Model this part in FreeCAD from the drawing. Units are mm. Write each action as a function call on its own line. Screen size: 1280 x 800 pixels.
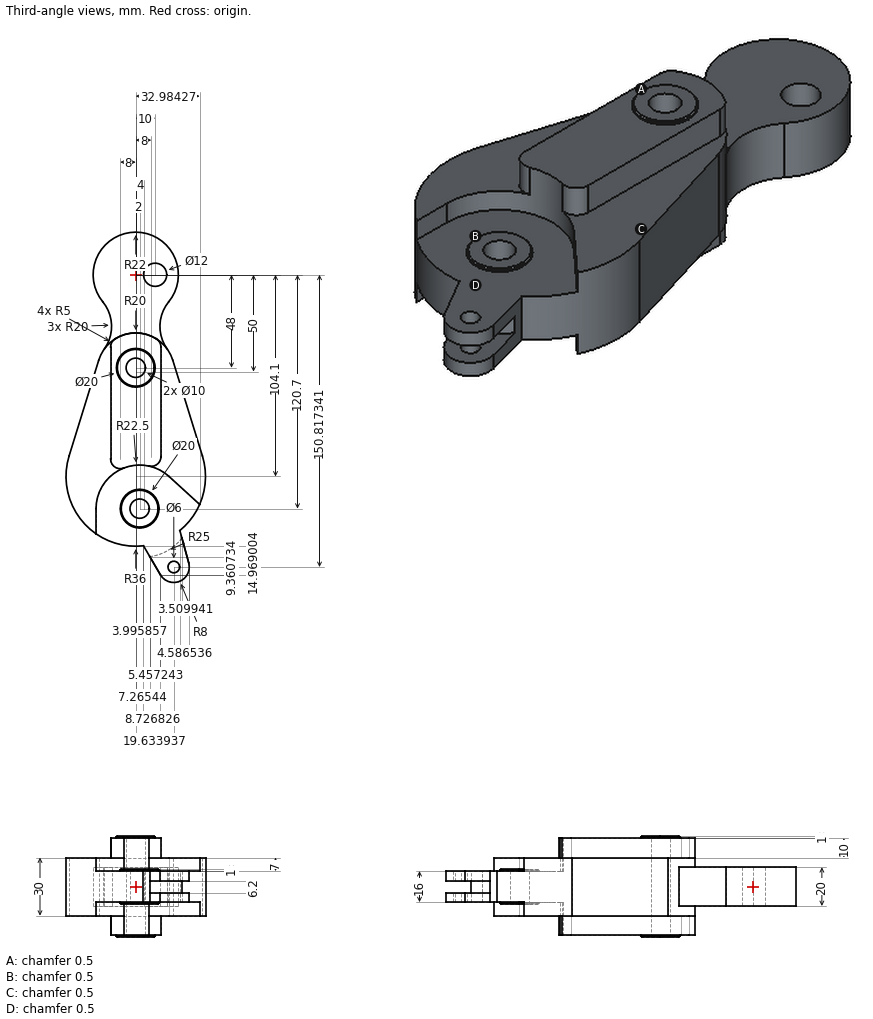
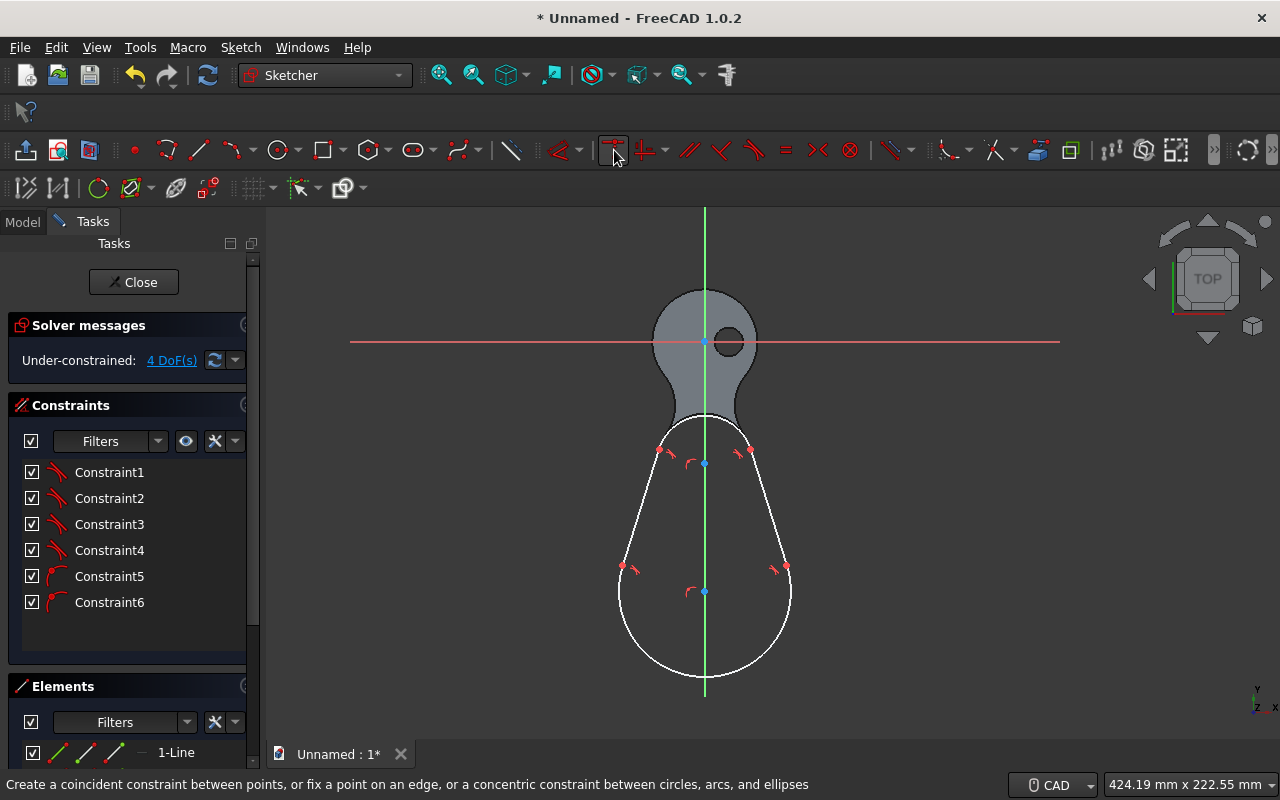
click(558, 150)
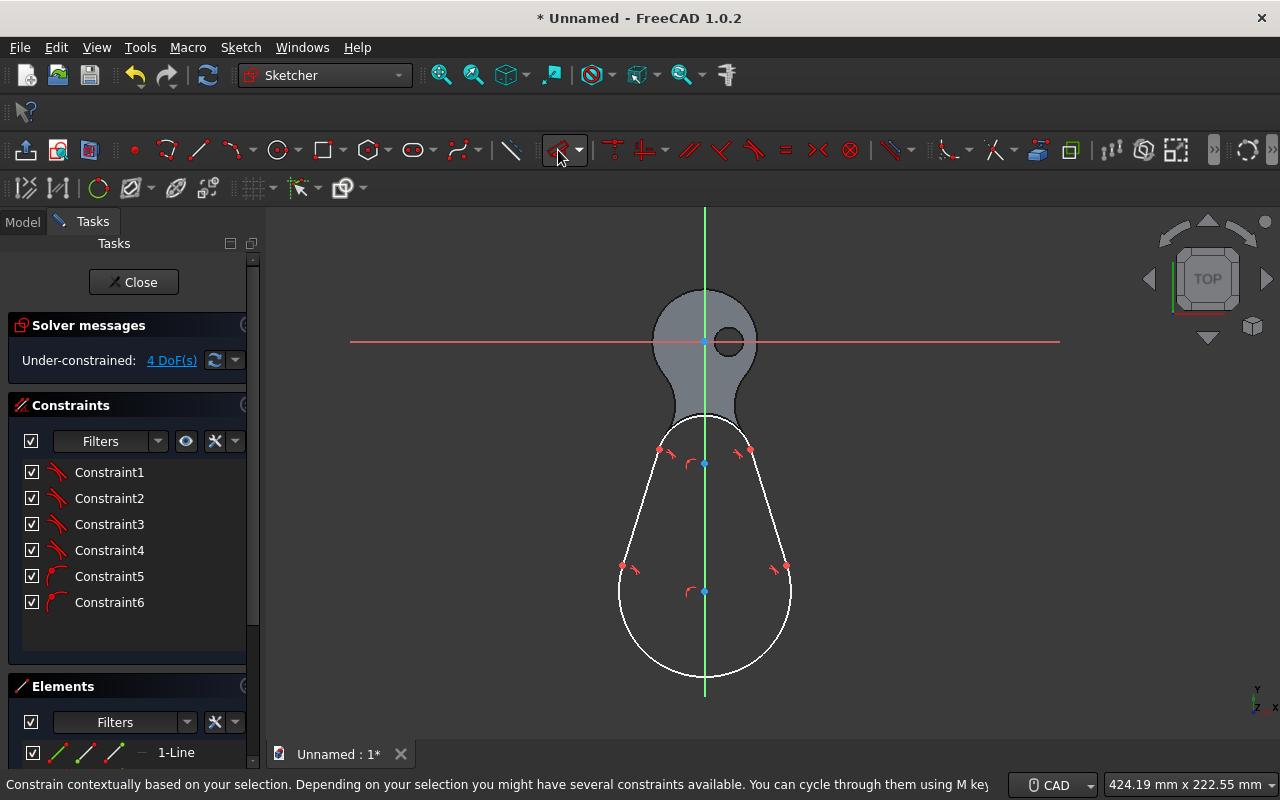
click(646, 654)
click(624, 677)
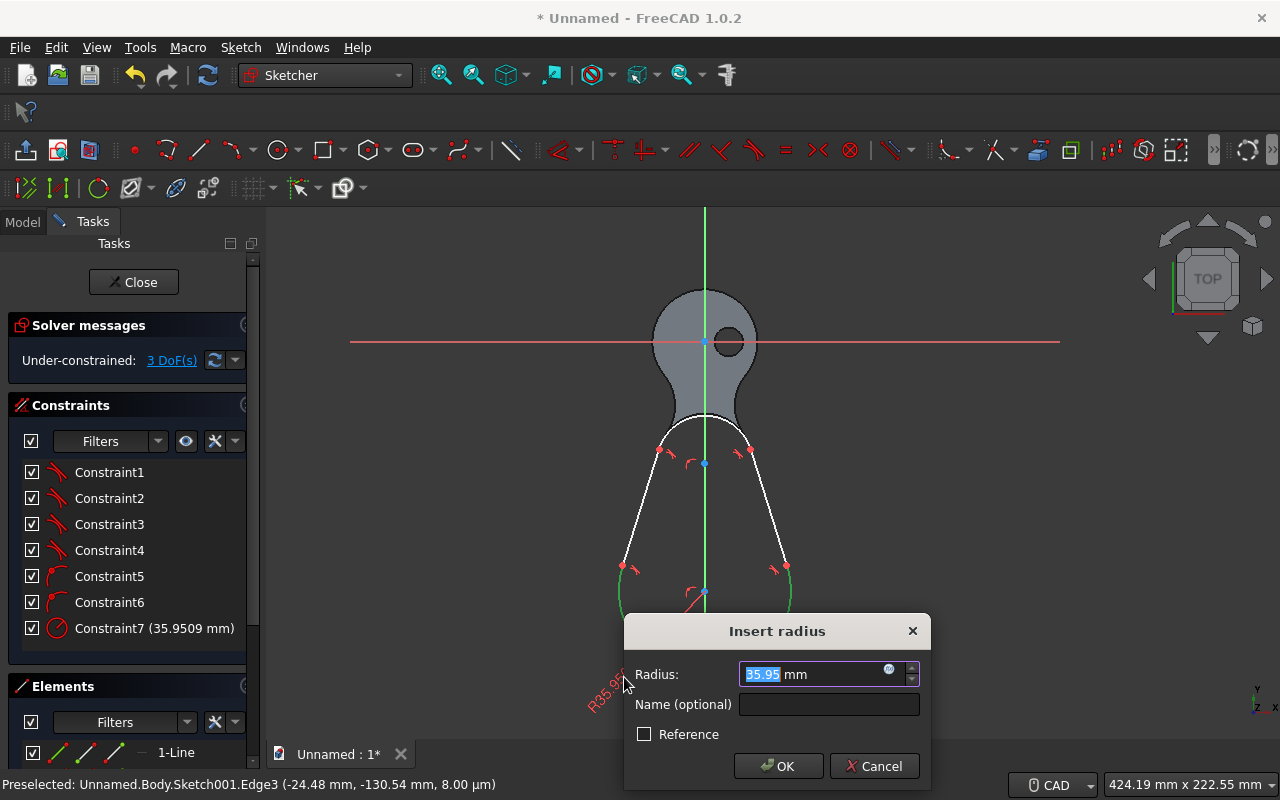
text(36)
key(Return)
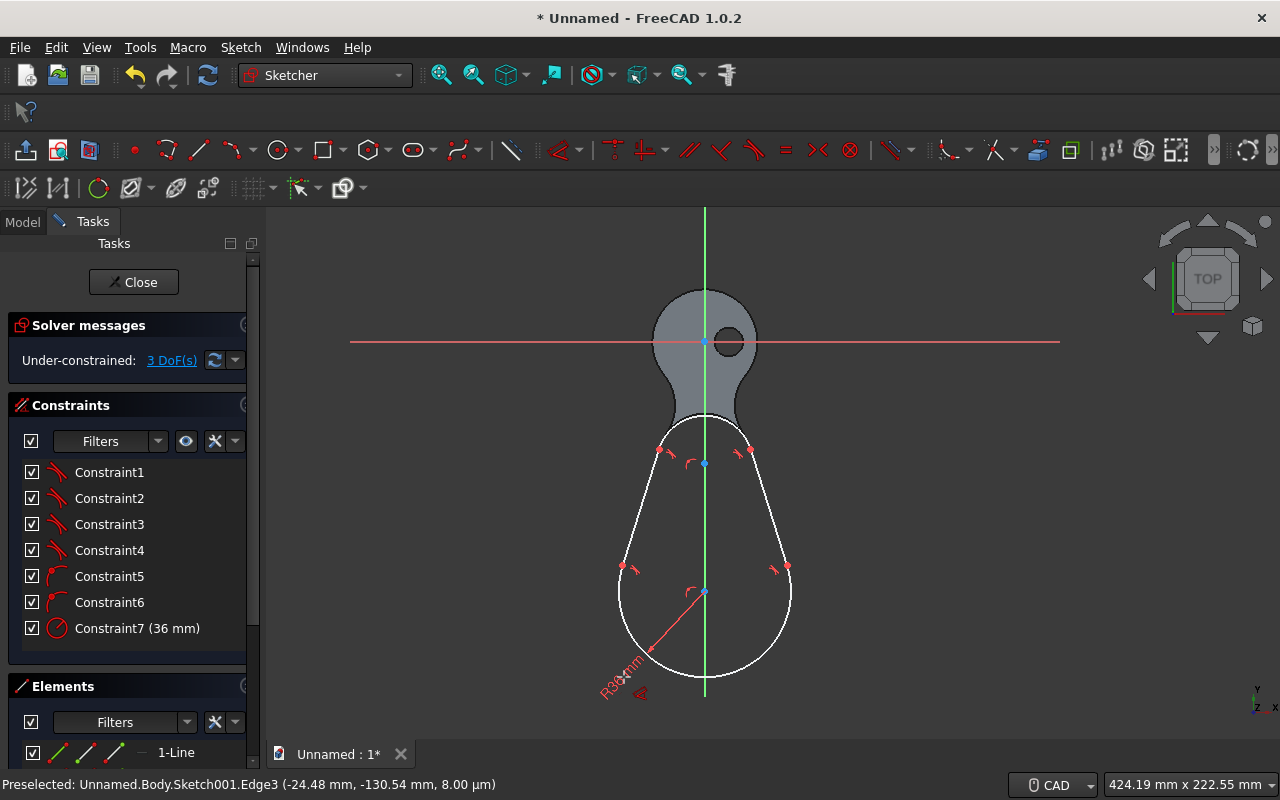
click(728, 422)
click(743, 394)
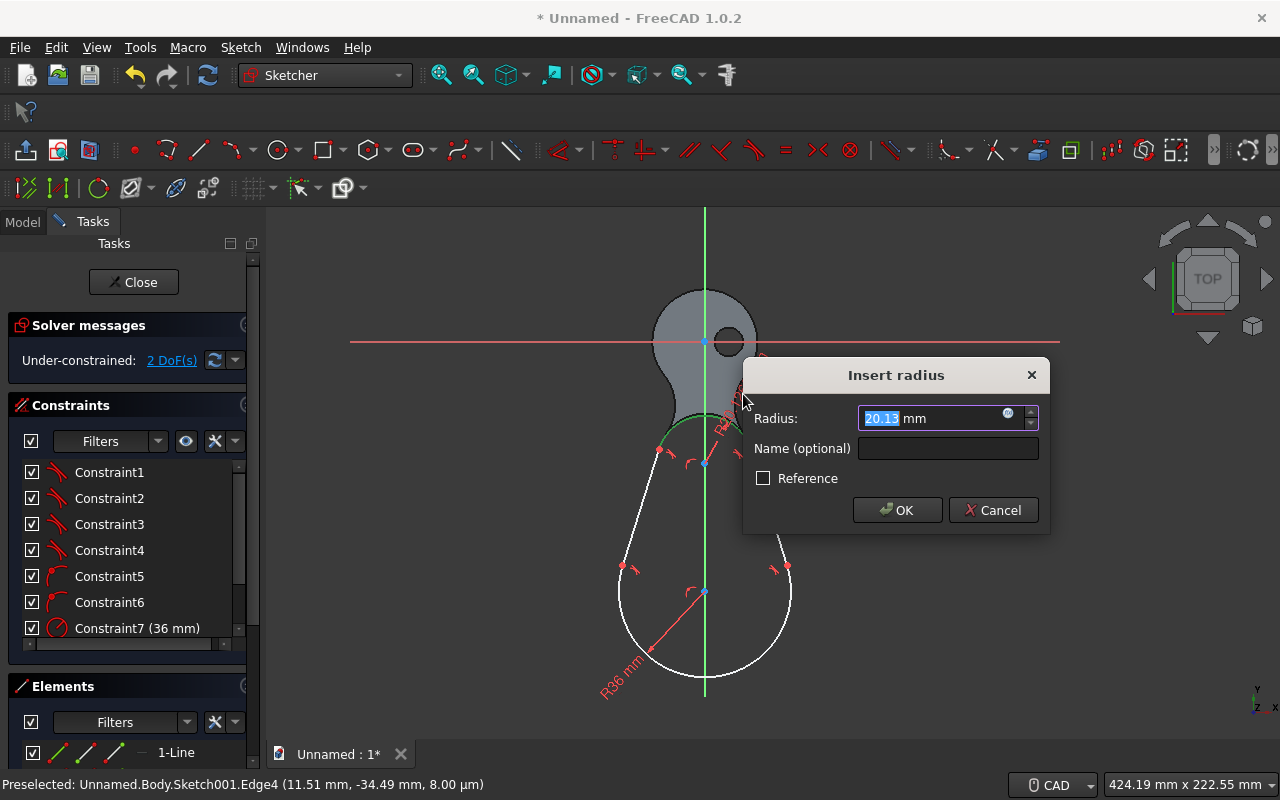
text(20)
key(Return)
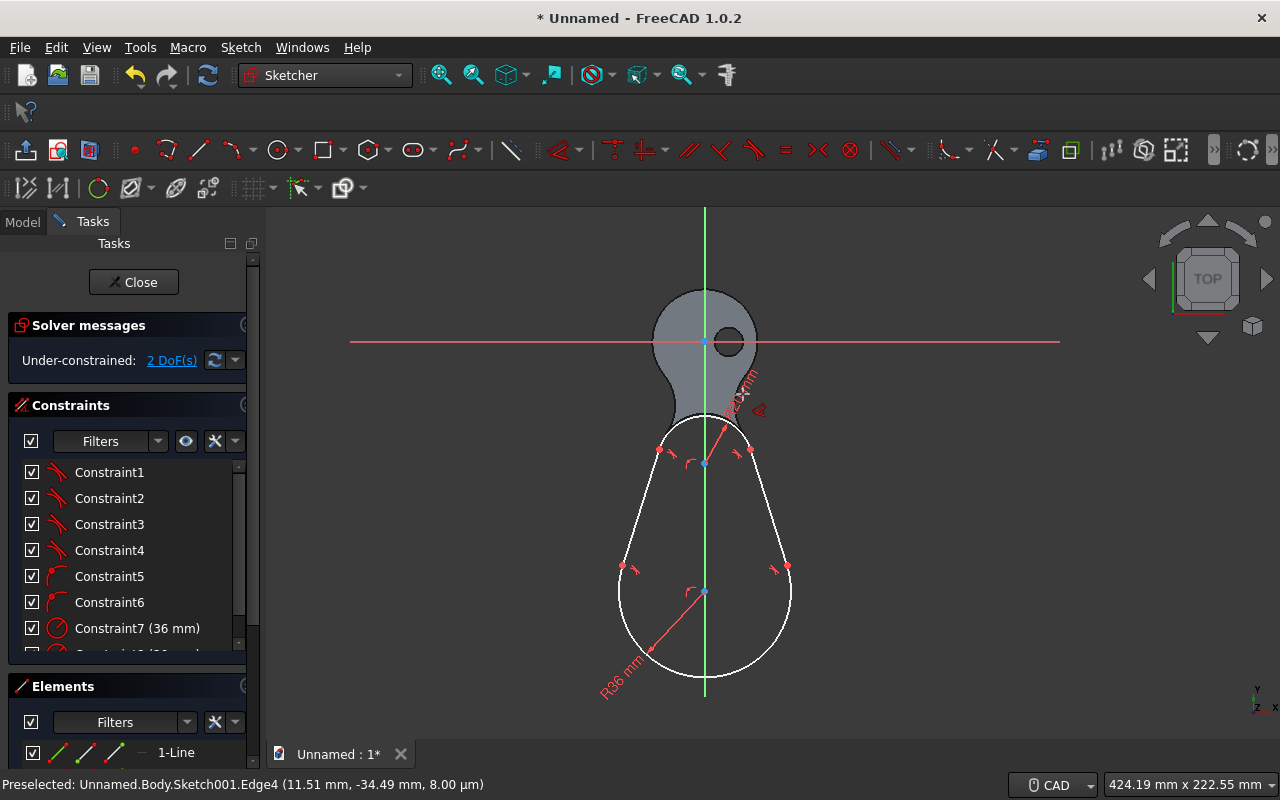
click(705, 464)
click(739, 360)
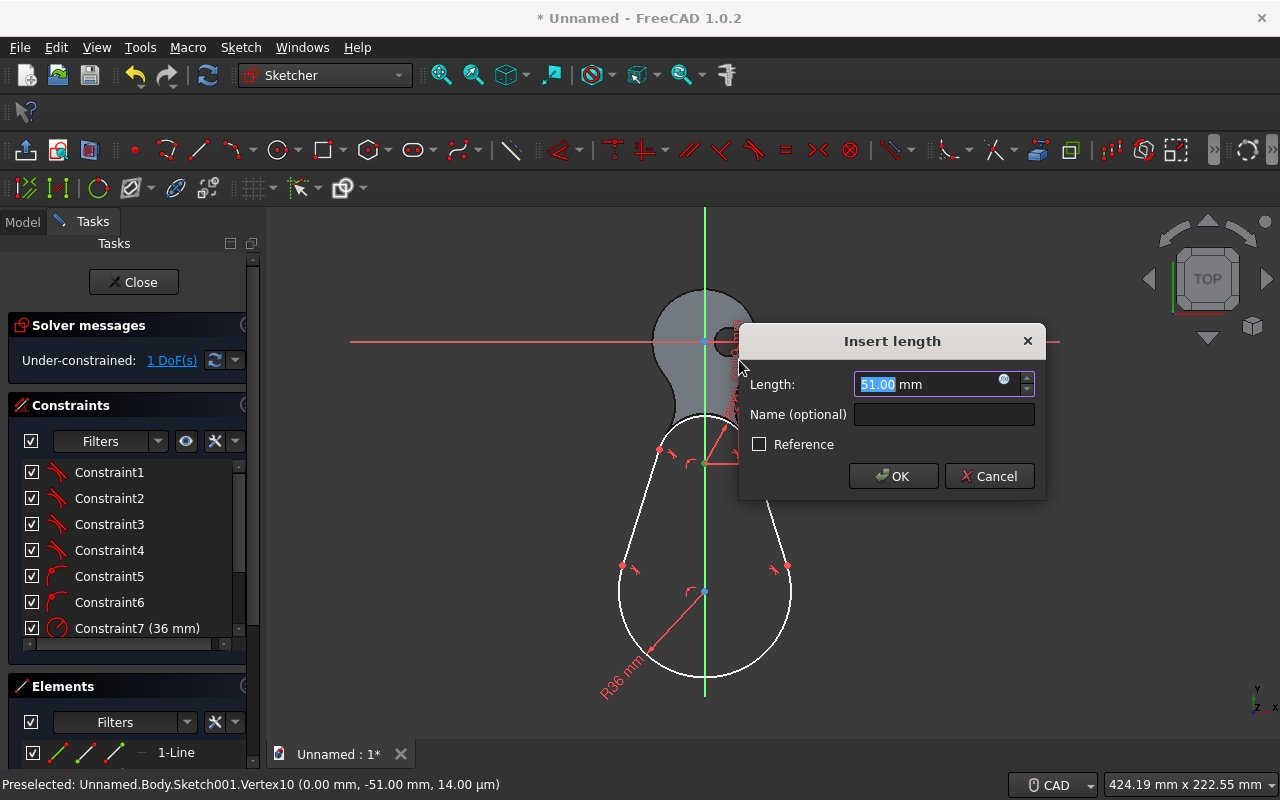
text(50)
key(Return)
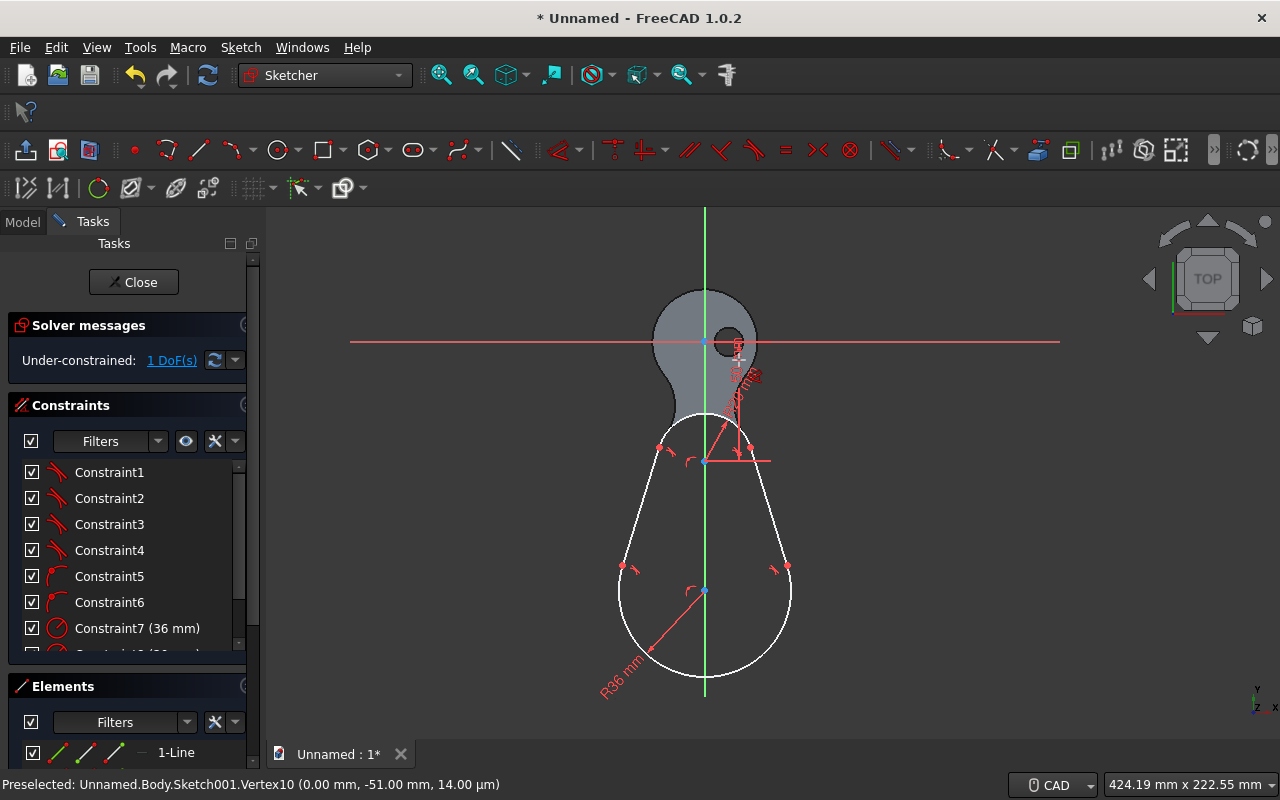
click(705, 591)
click(739, 466)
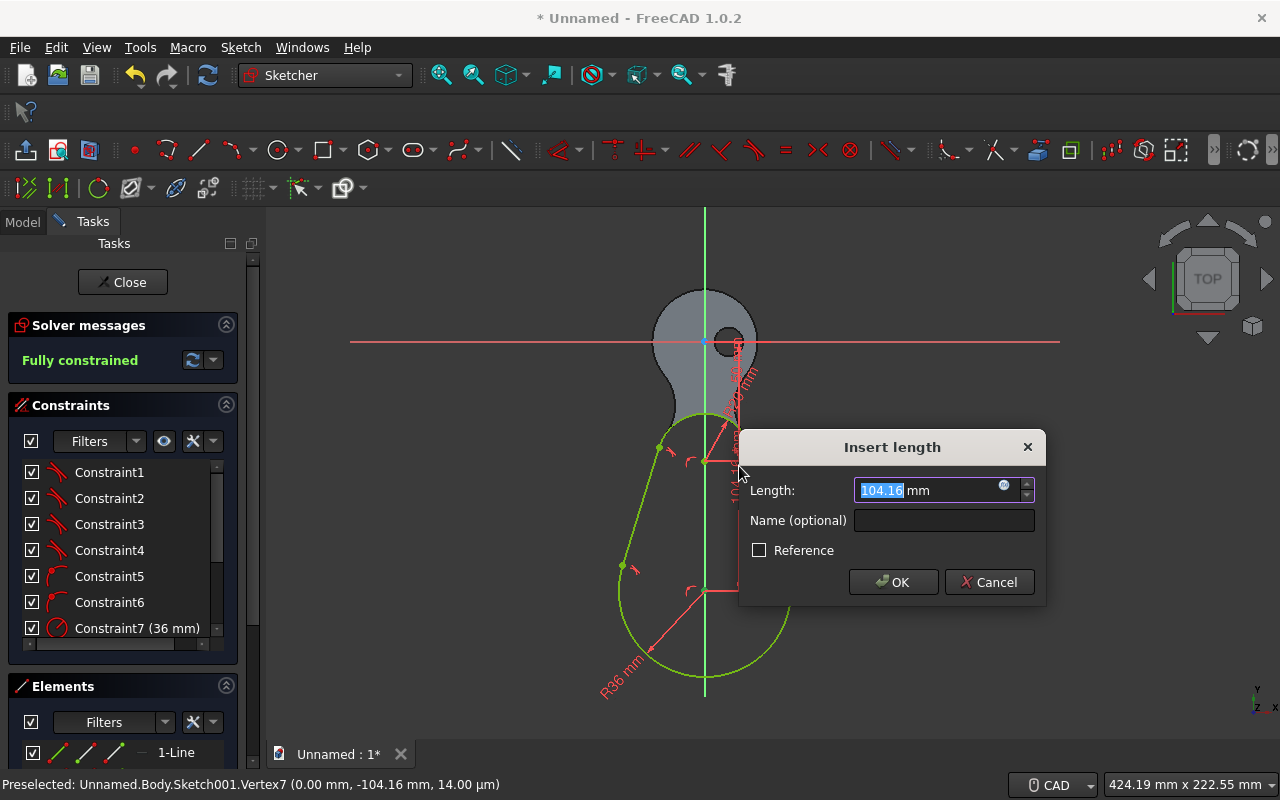
text(104.1)
key(Return)
key(Escape)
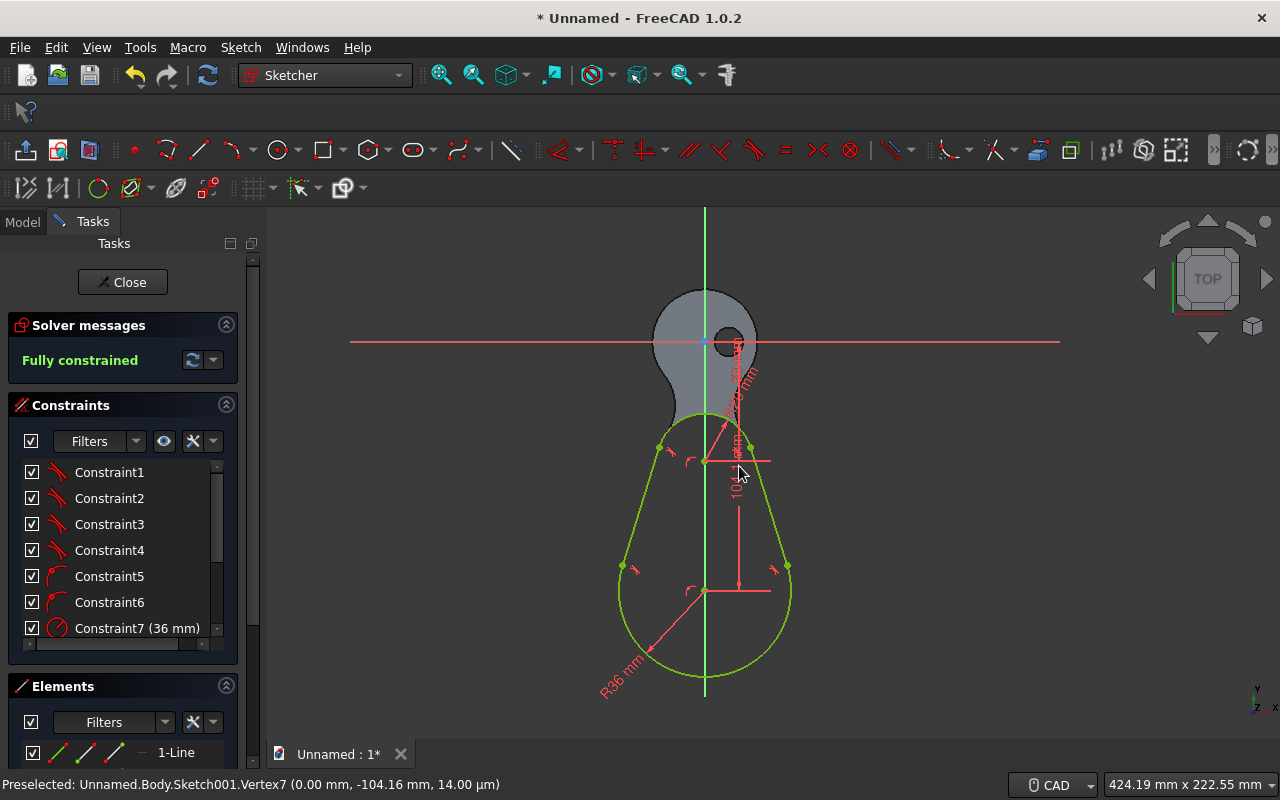
click(123, 282)